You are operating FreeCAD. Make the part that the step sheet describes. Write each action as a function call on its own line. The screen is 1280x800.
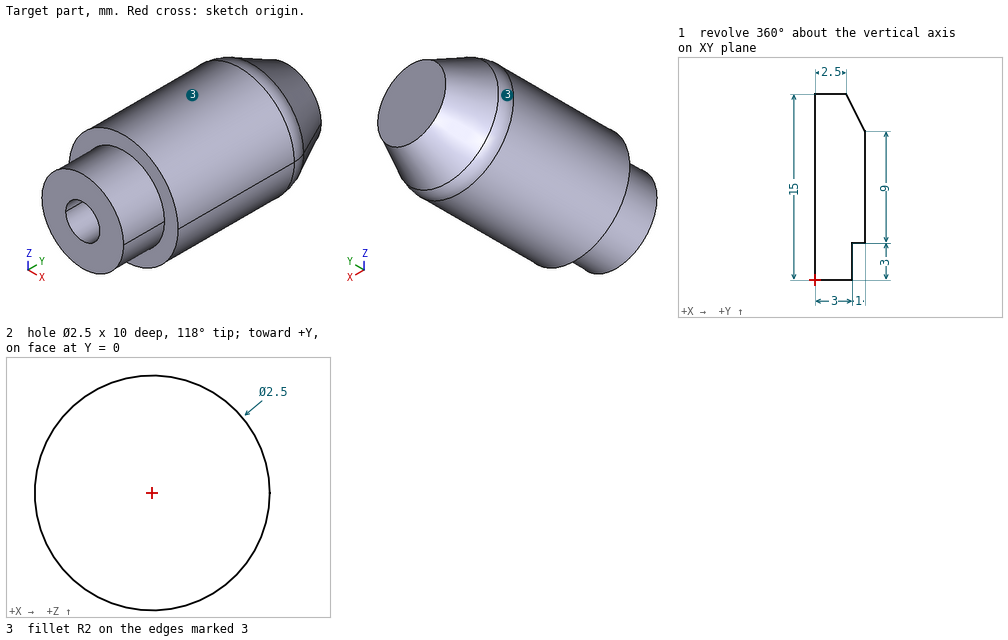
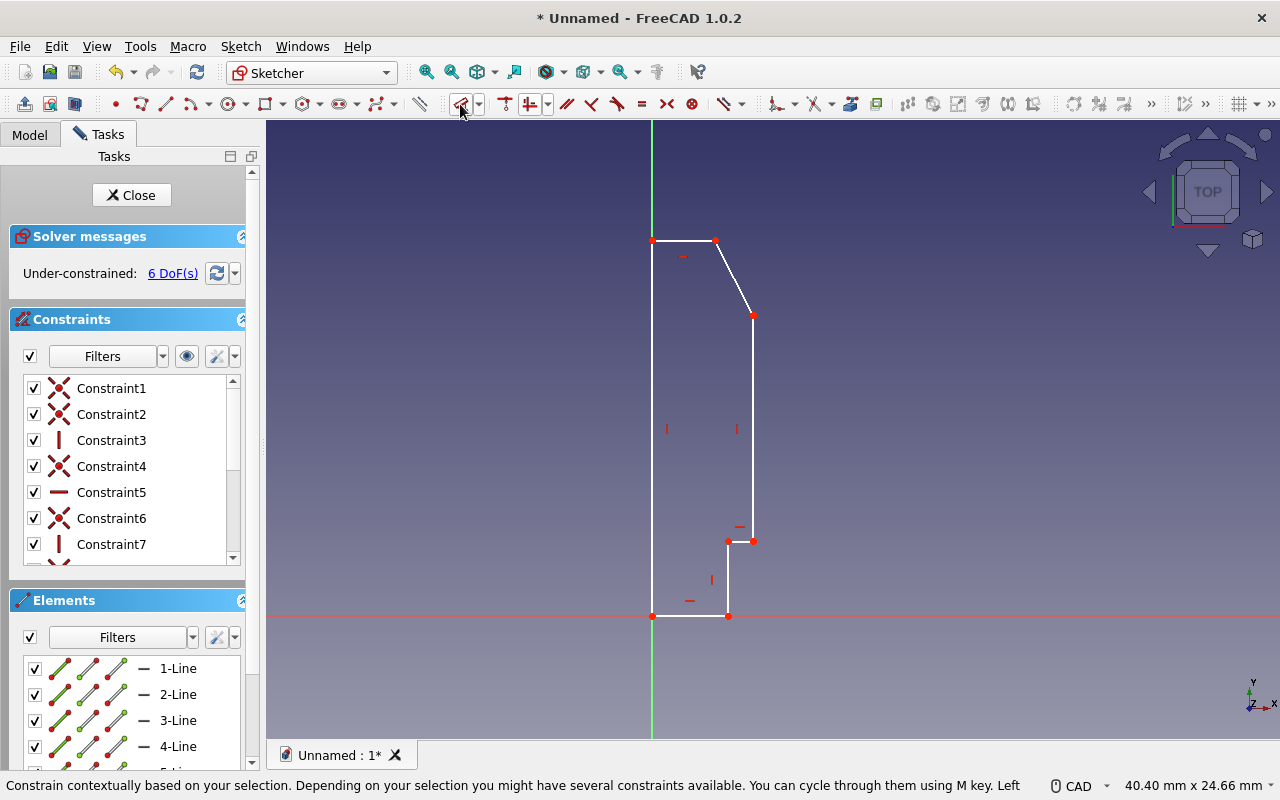
click(675, 616)
click(690, 650)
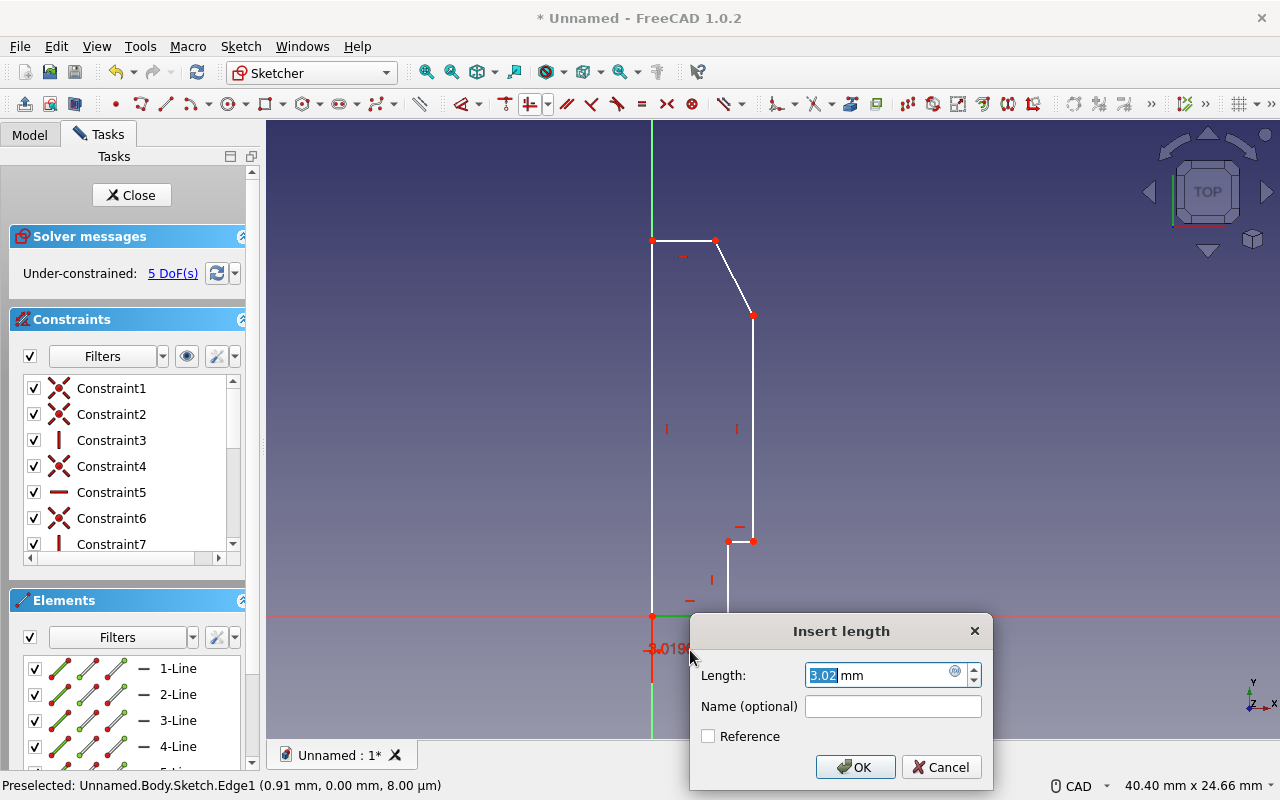
text(3)
key(Return)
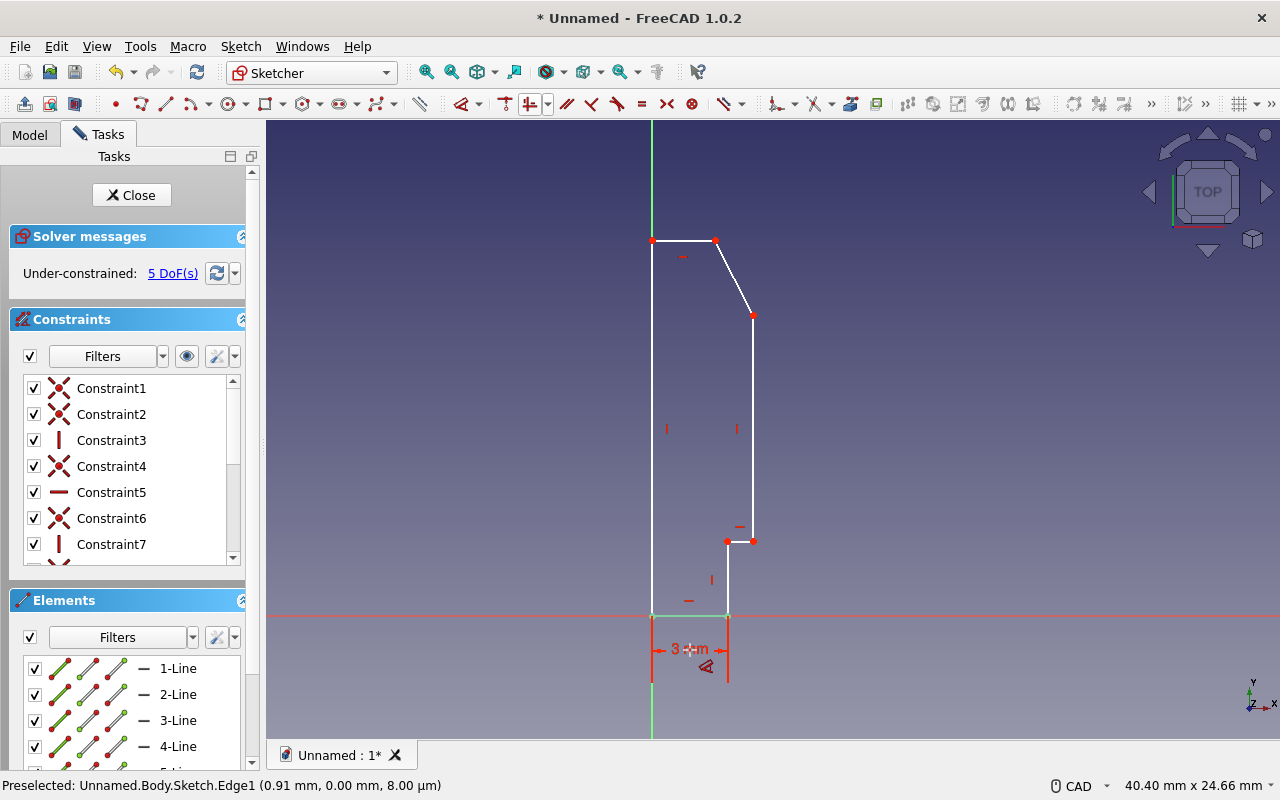
click(728, 594)
click(762, 579)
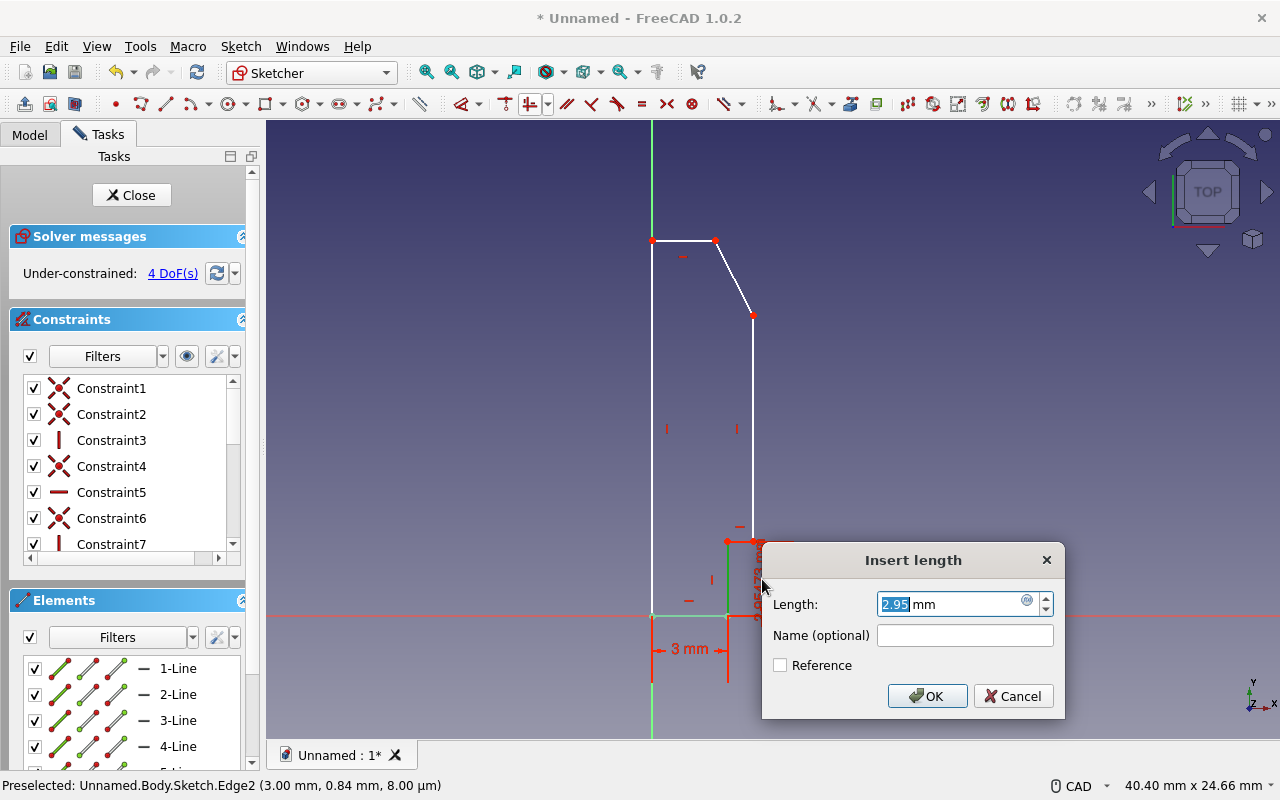
text(3)
key(Return)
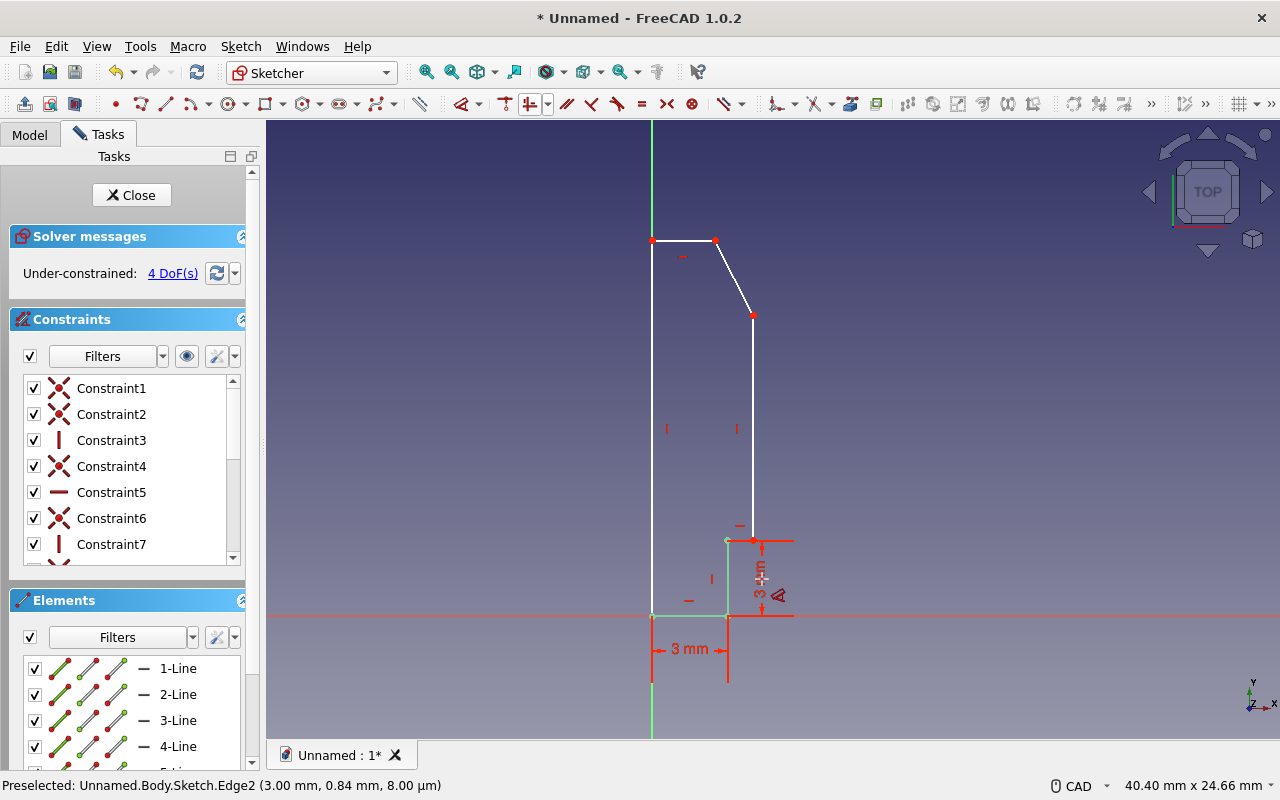
scroll(738, 541, up, 3)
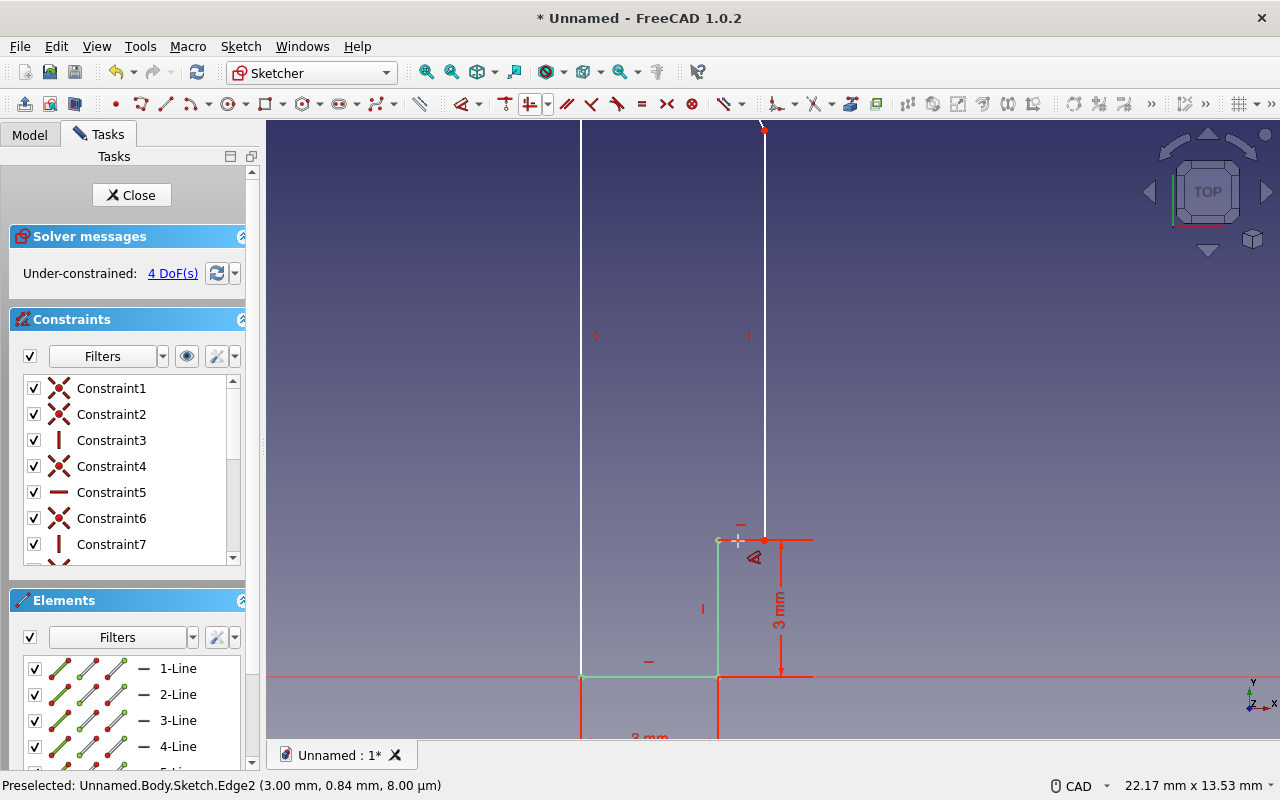
click(737, 540)
click(742, 574)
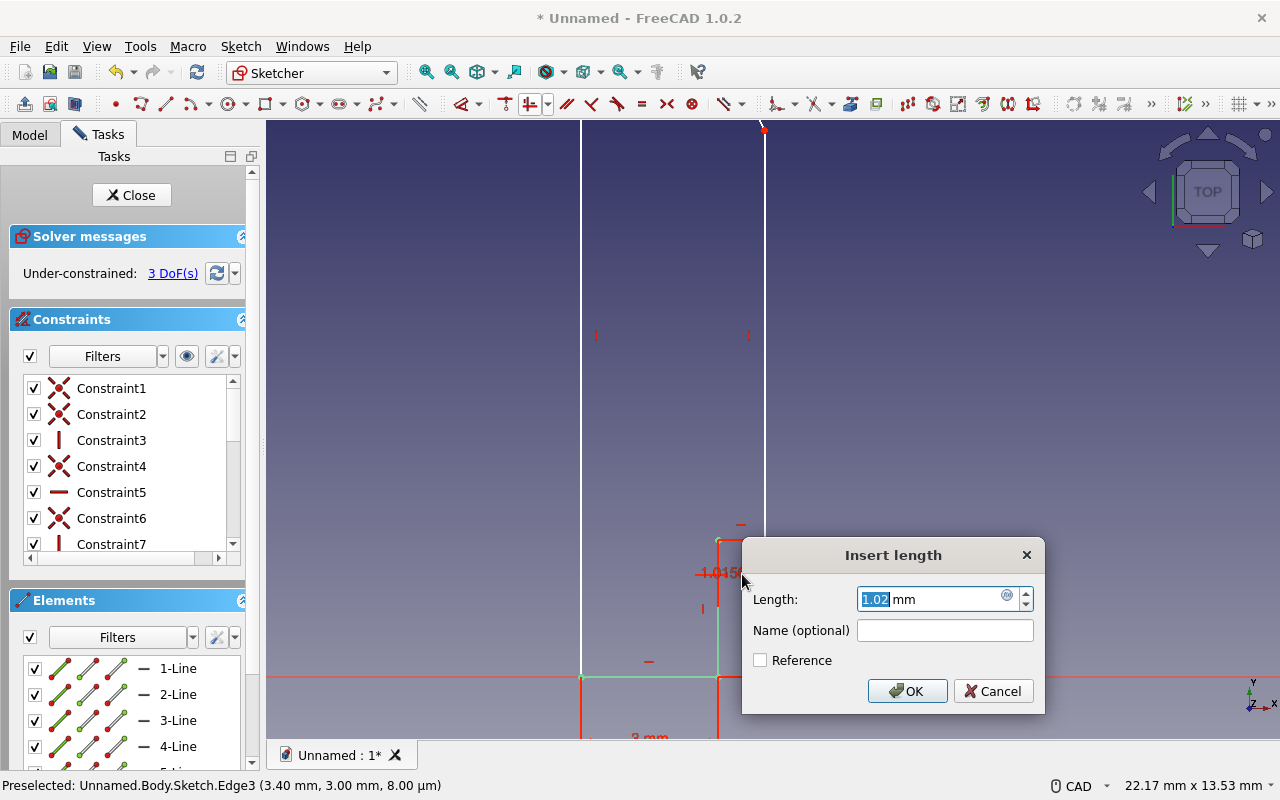
text(1)
key(Return)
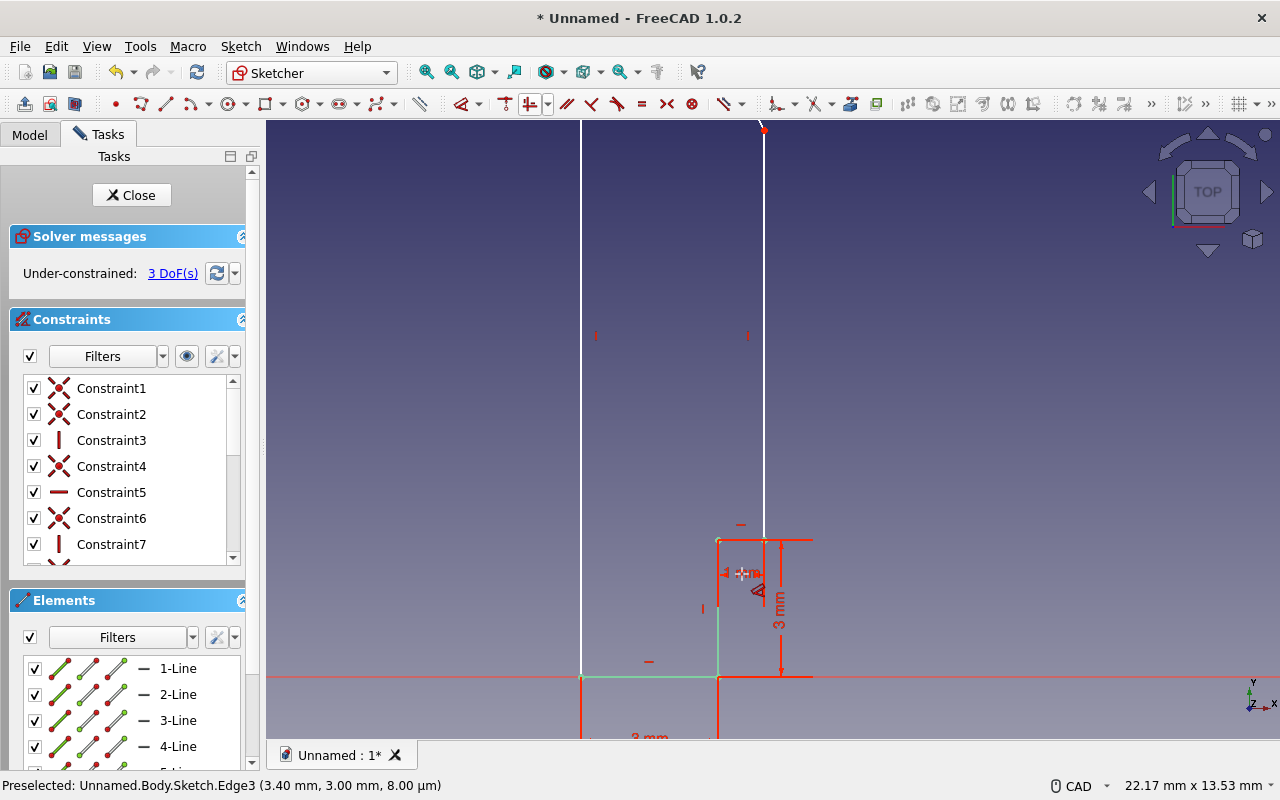
click(764, 417)
click(798, 344)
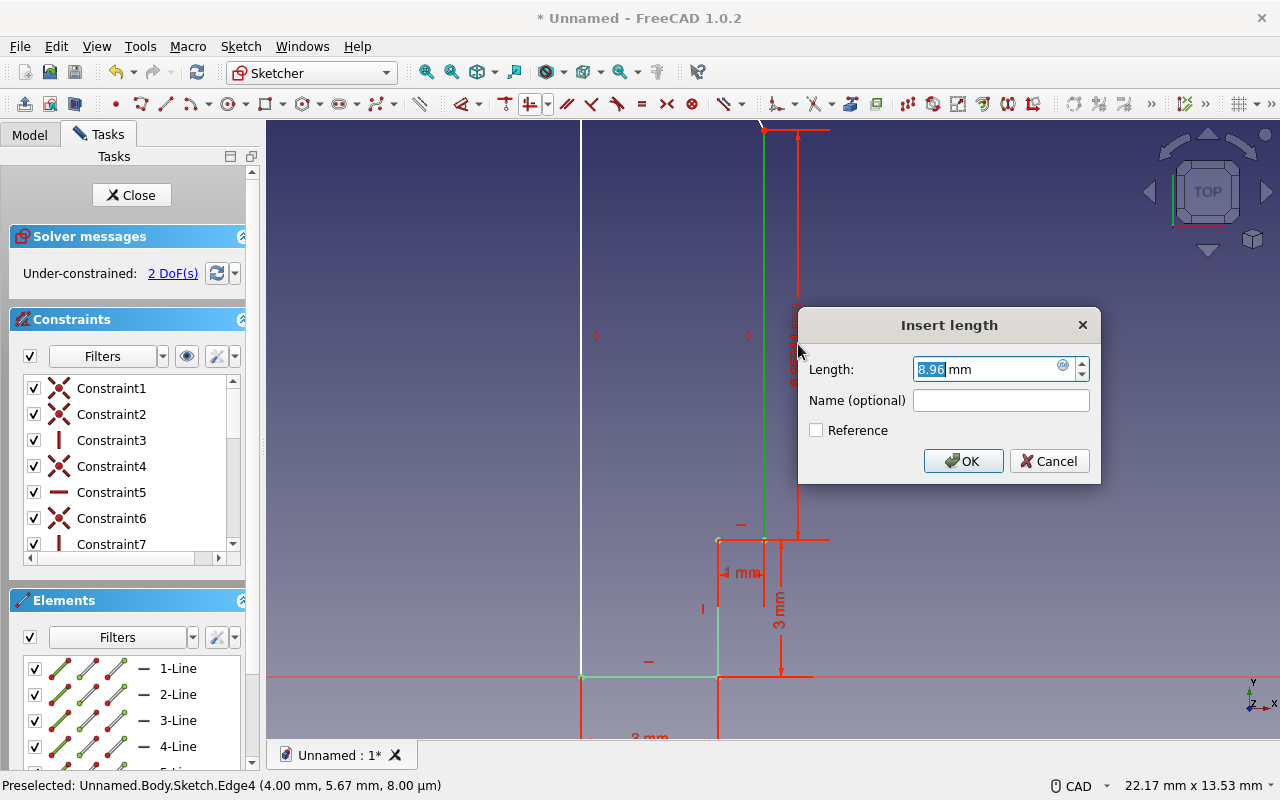
text(9)
key(Return)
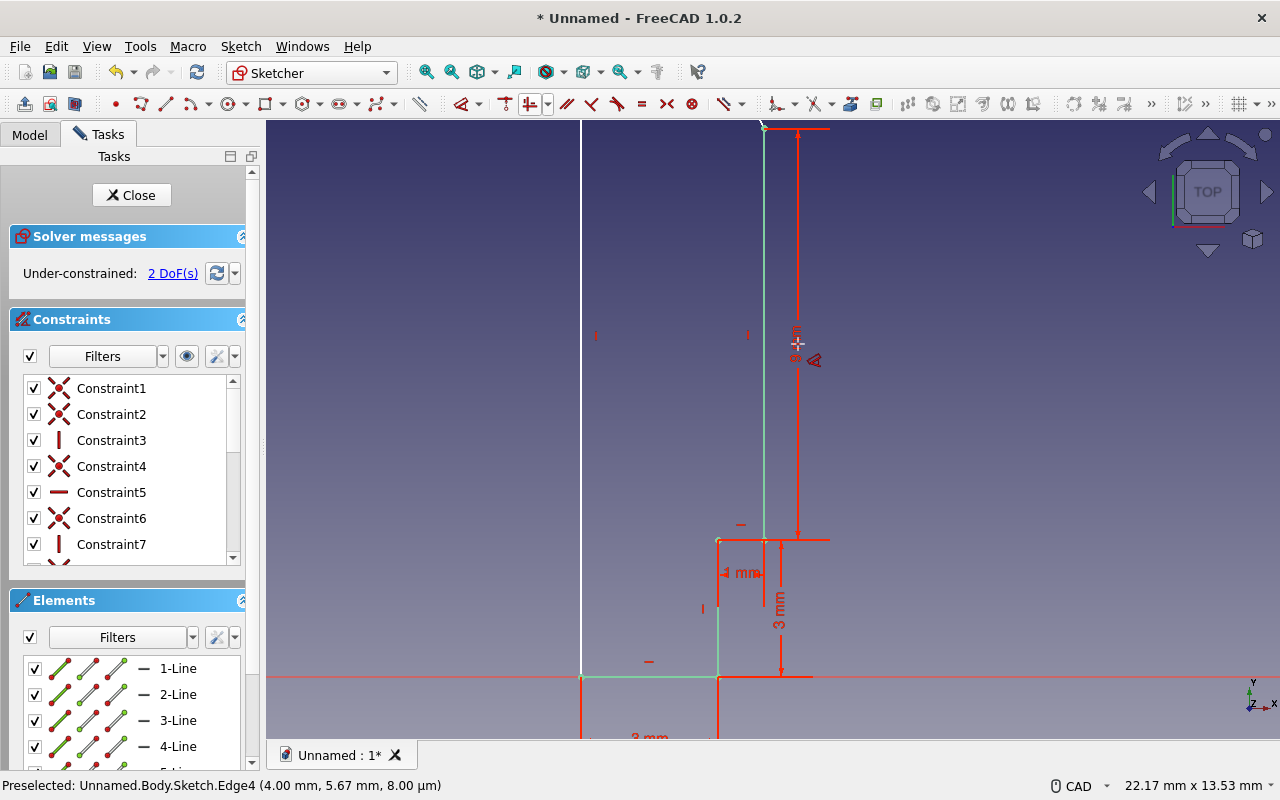
click(581, 199)
click(547, 413)